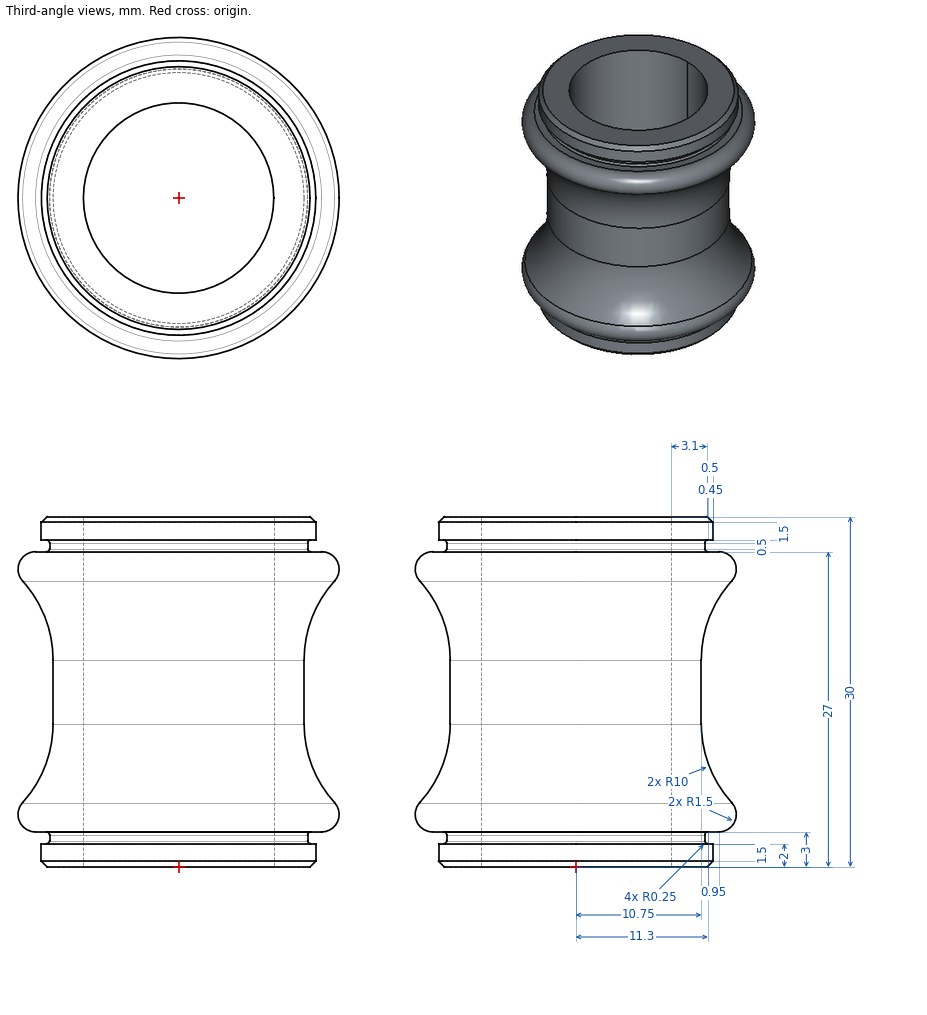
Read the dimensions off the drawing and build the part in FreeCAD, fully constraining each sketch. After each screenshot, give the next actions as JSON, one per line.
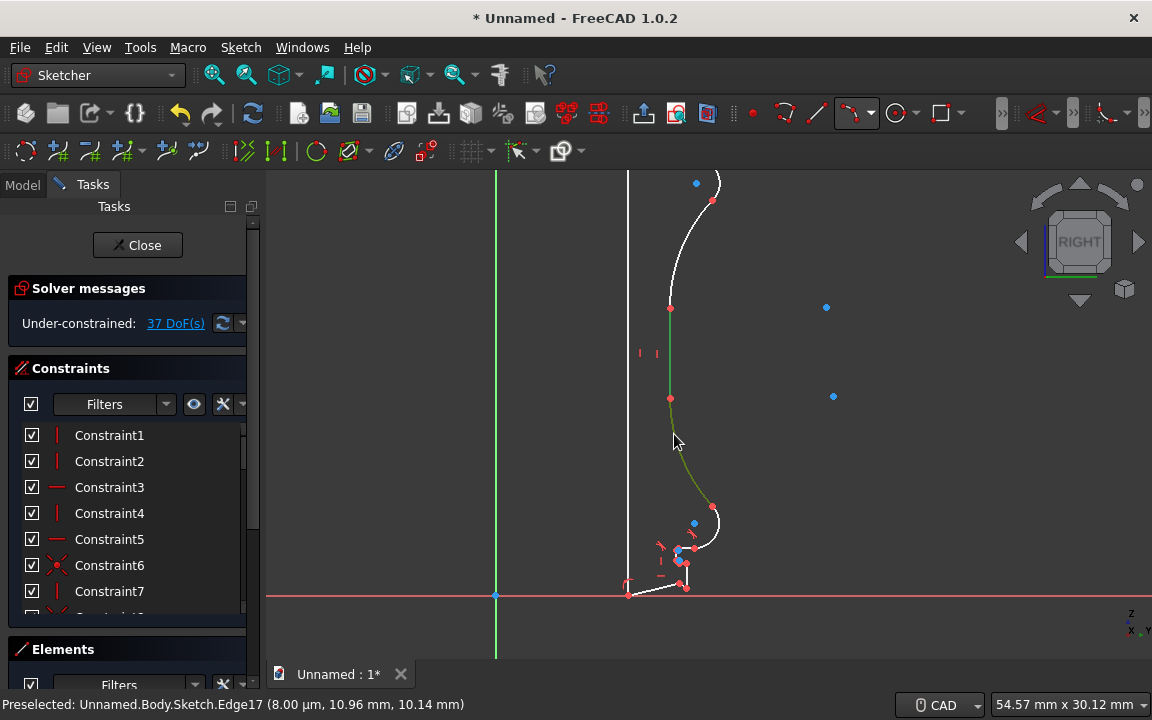
{"action": "key", "text": "t"}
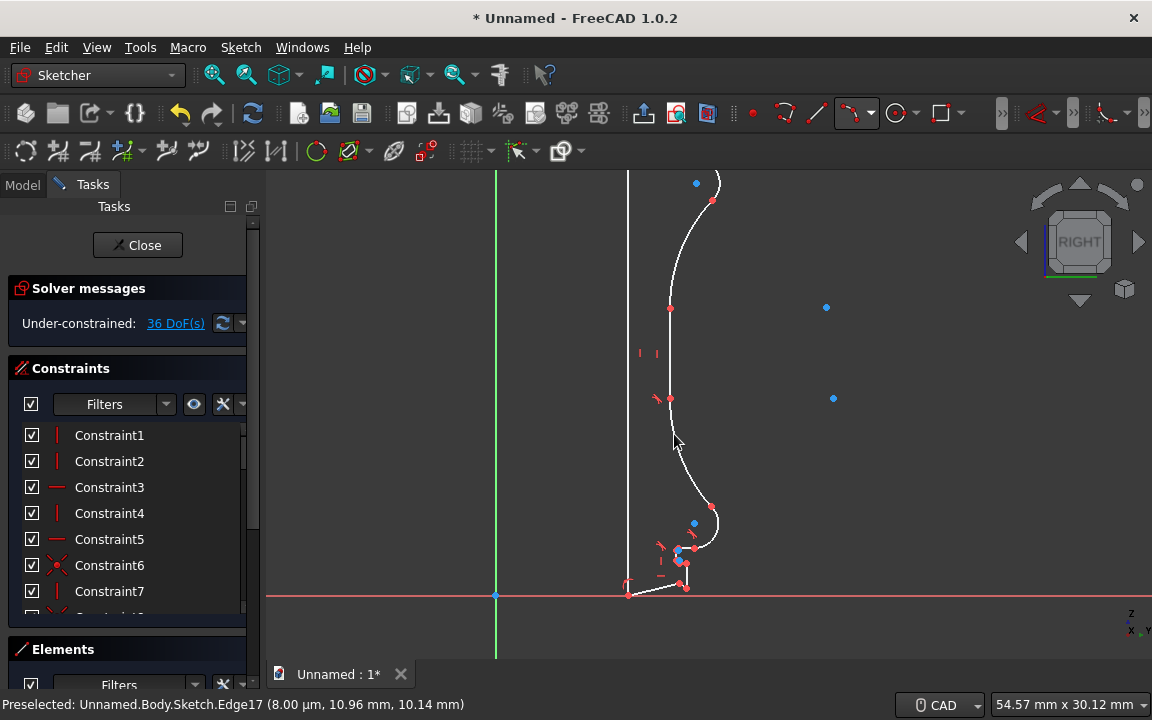
{"action": "left_click", "coordinate": [670, 371]}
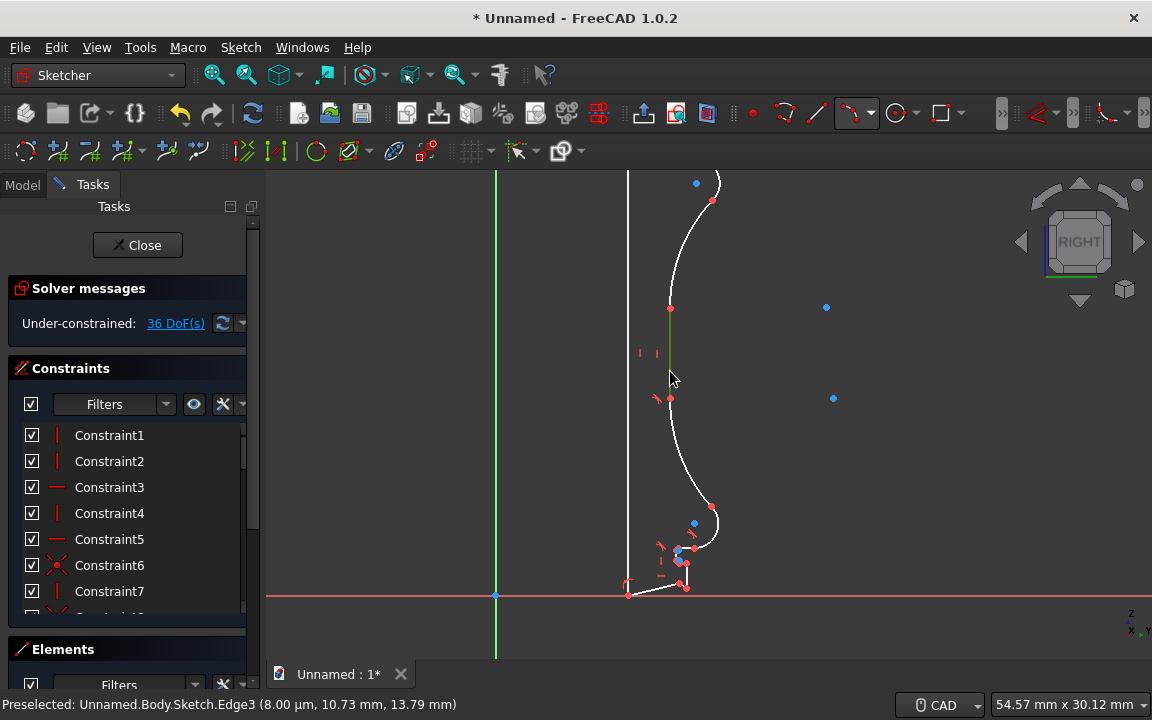
{"action": "left_click", "coordinate": [691, 229]}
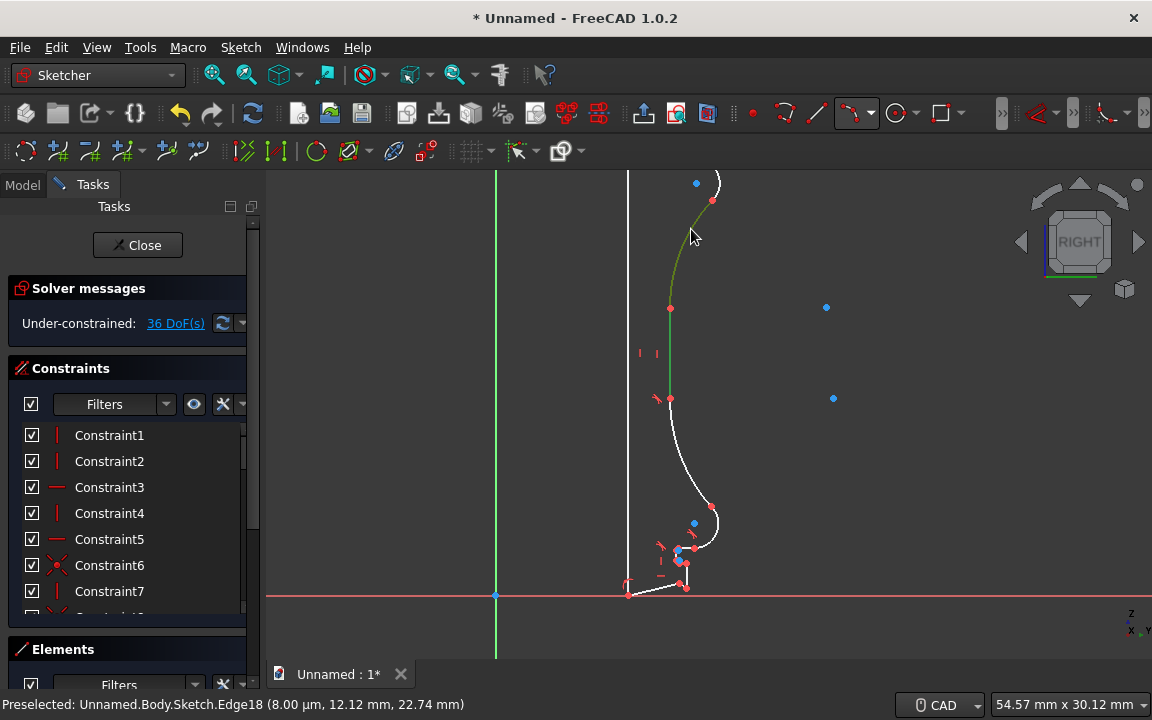
{"action": "key", "text": "t"}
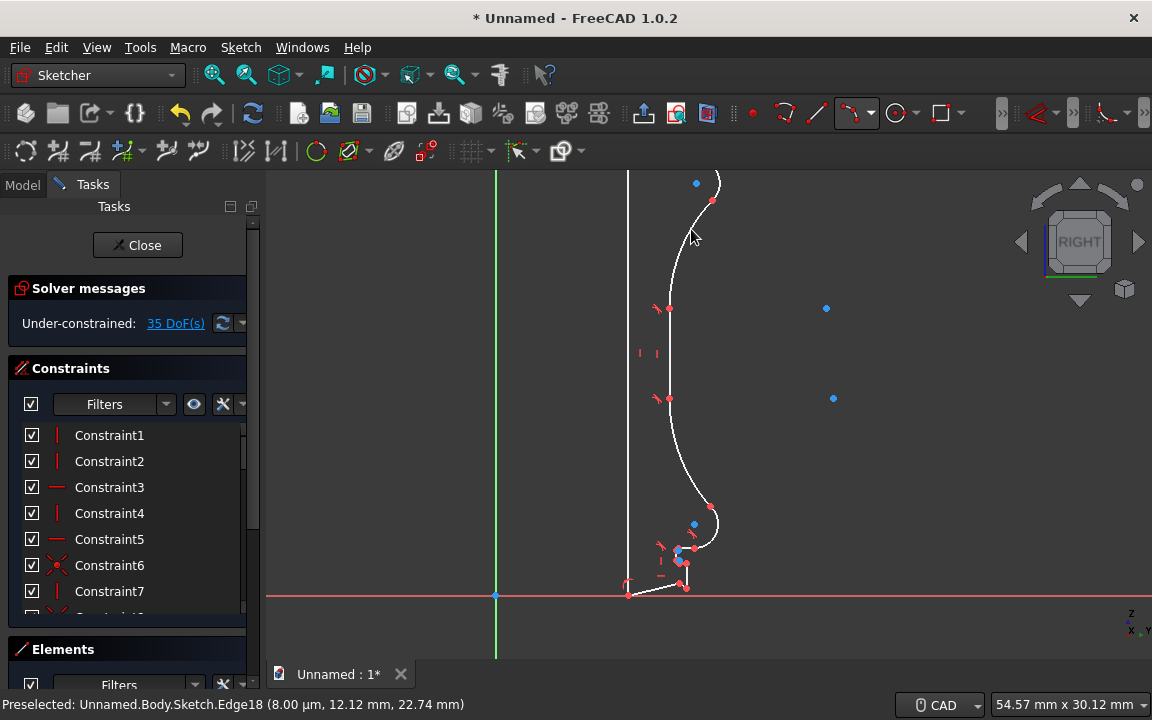
{"action": "scroll", "coordinate": [710, 541], "scroll_direction": "down", "scroll_amount": 2}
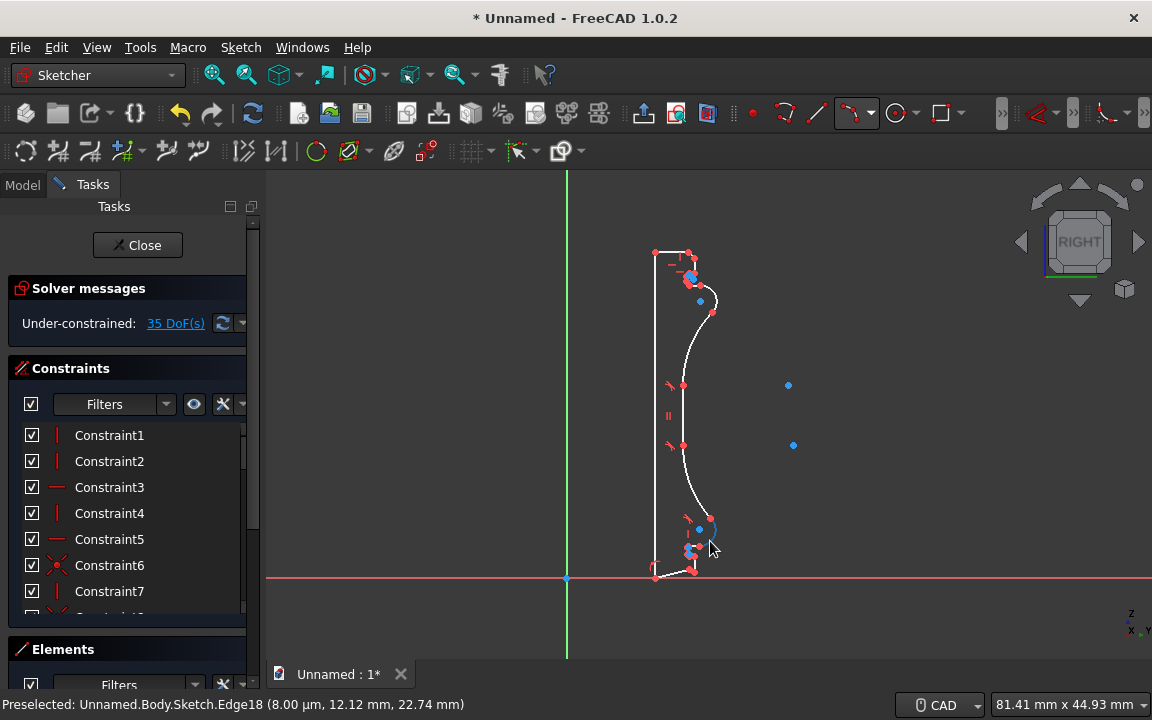
{"action": "scroll", "coordinate": [695, 286], "scroll_direction": "up", "scroll_amount": 5}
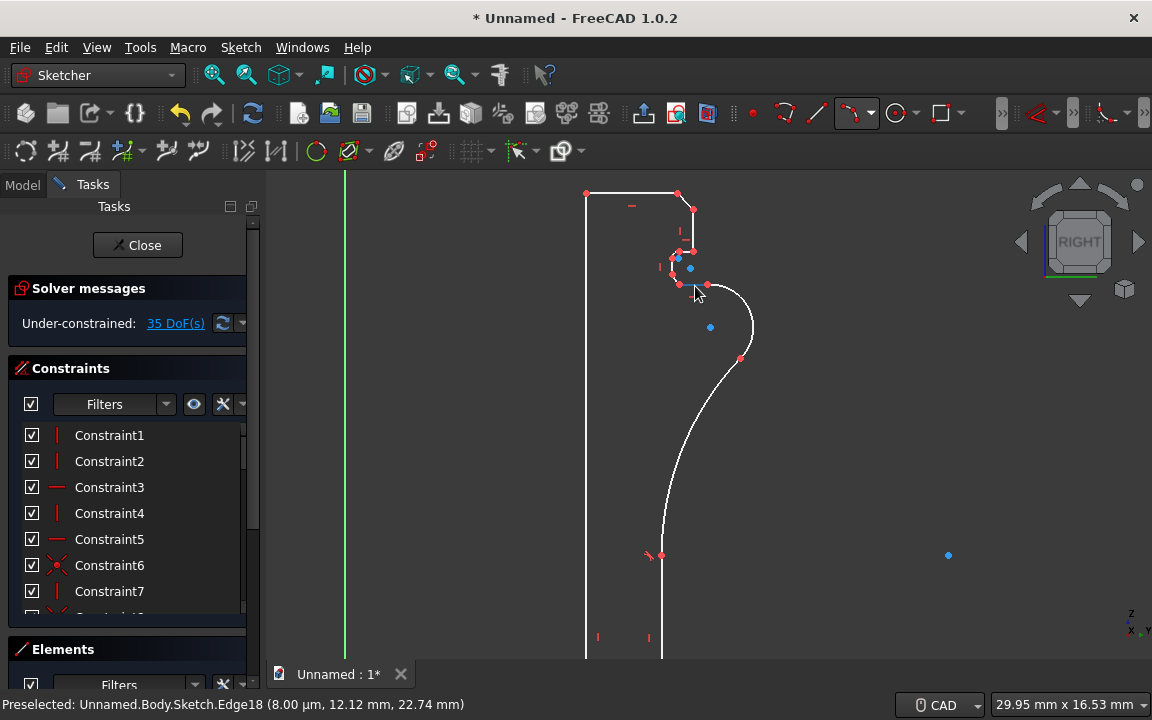
{"action": "left_click", "coordinate": [694, 285]}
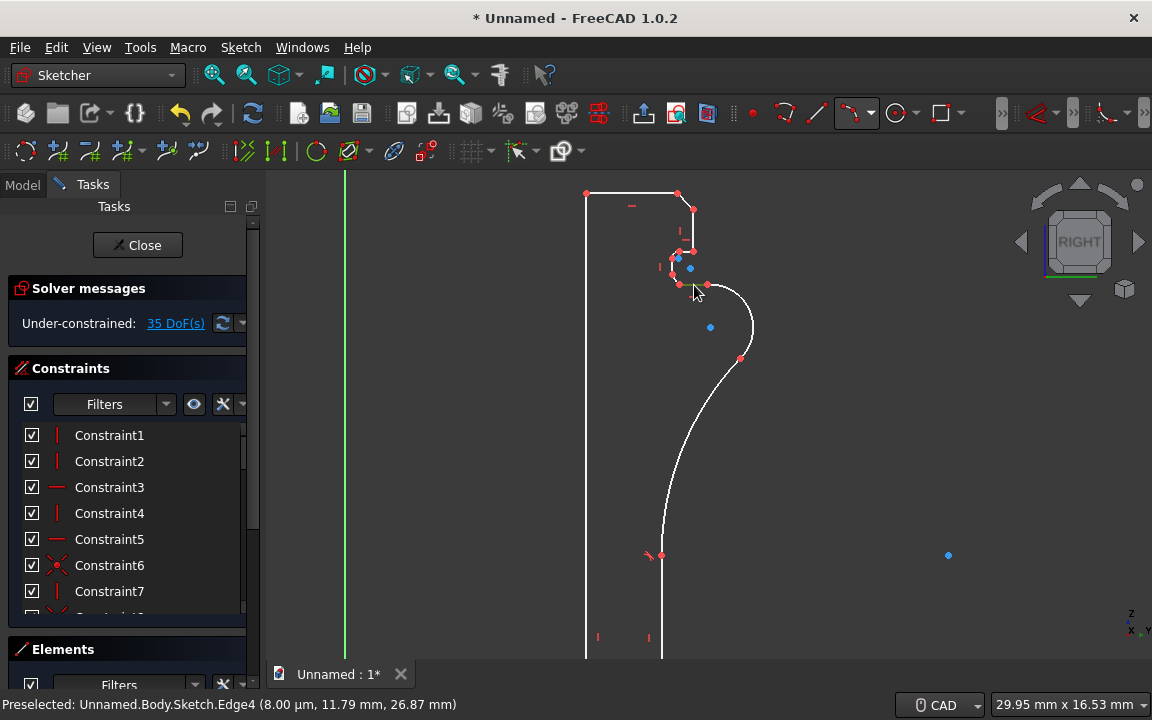
{"action": "left_click", "coordinate": [753, 330]}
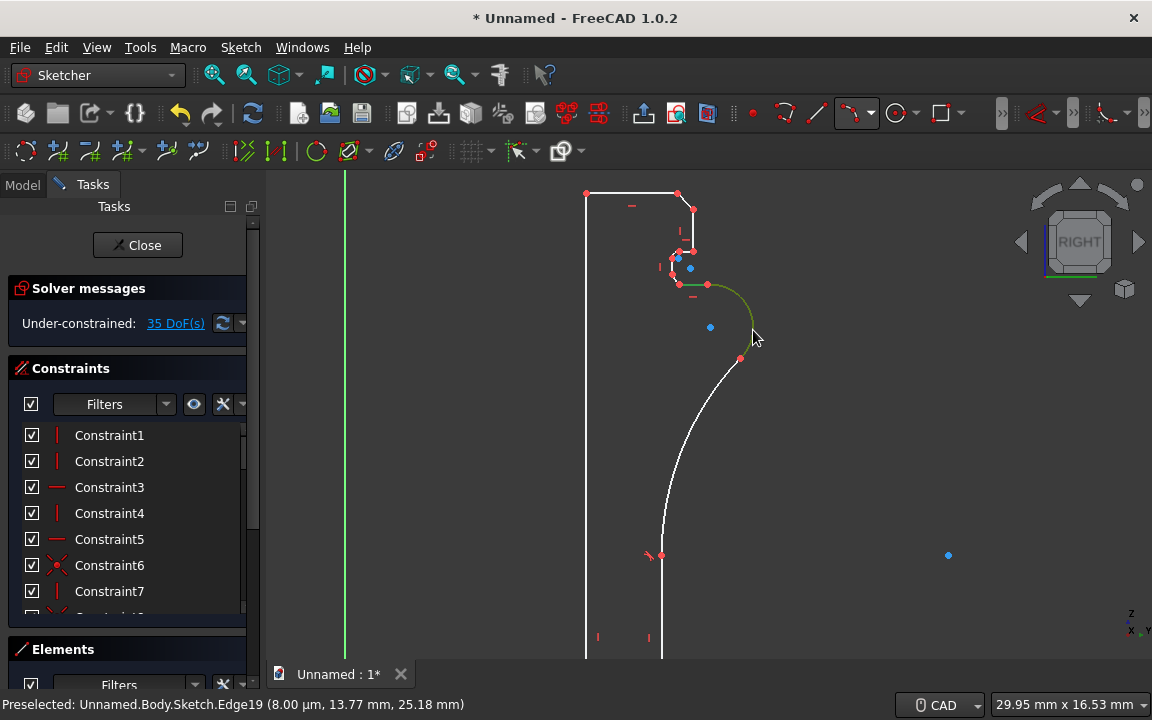
{"action": "key", "text": "t"}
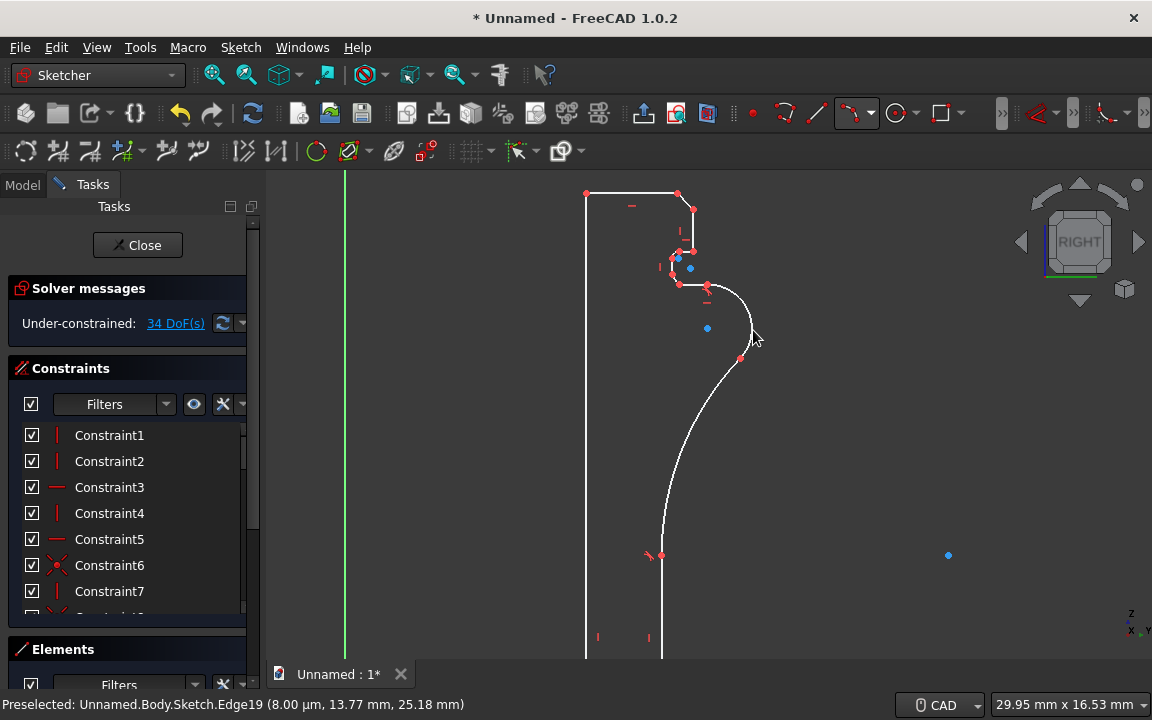
{"action": "scroll", "coordinate": [697, 285], "scroll_direction": "up", "scroll_amount": 2}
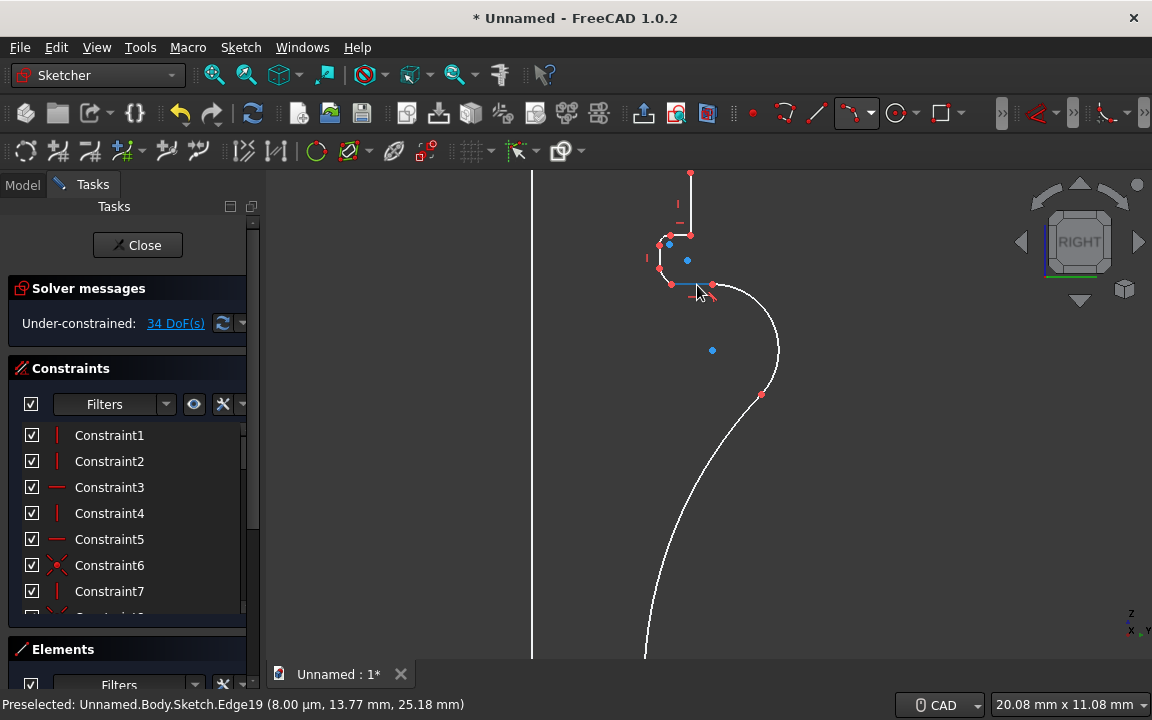
{"action": "left_click", "coordinate": [696, 284]}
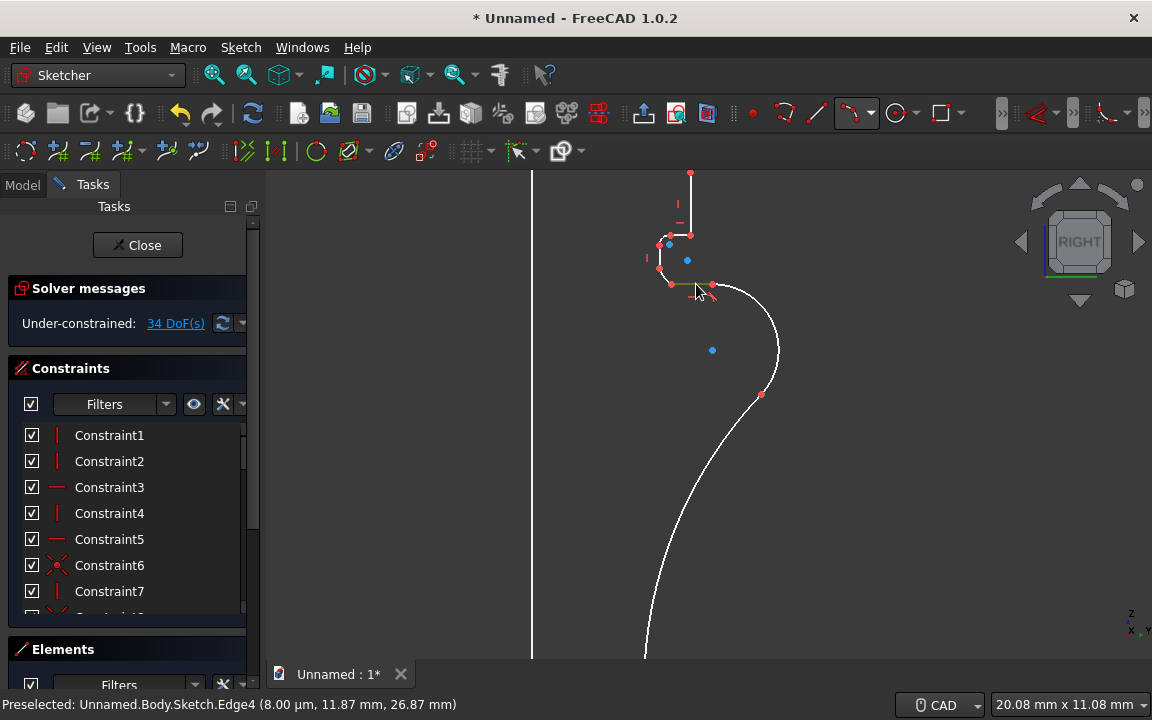
{"action": "scroll", "coordinate": [664, 277], "scroll_direction": "up", "scroll_amount": 2}